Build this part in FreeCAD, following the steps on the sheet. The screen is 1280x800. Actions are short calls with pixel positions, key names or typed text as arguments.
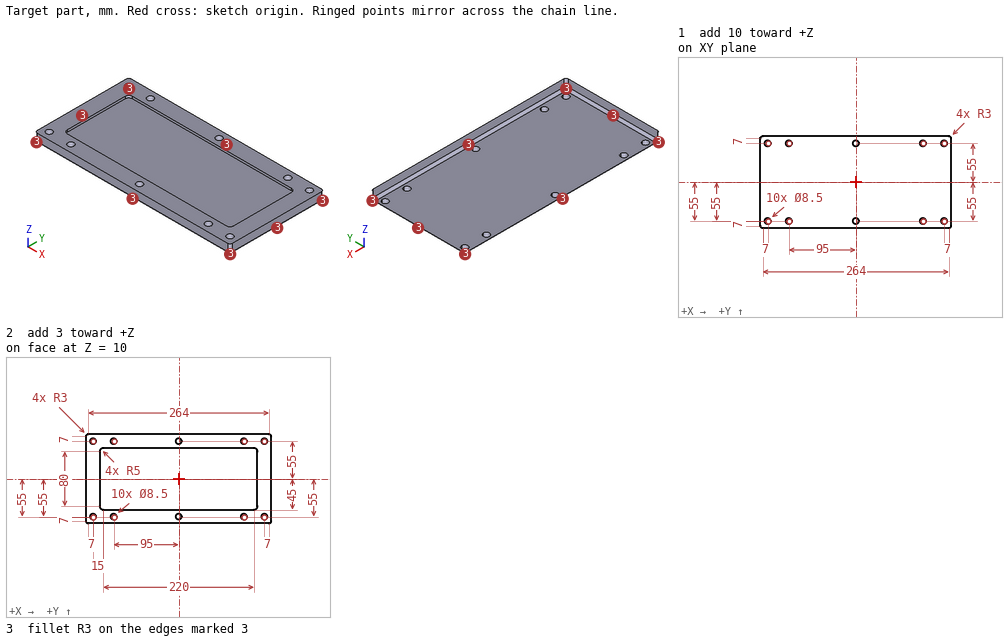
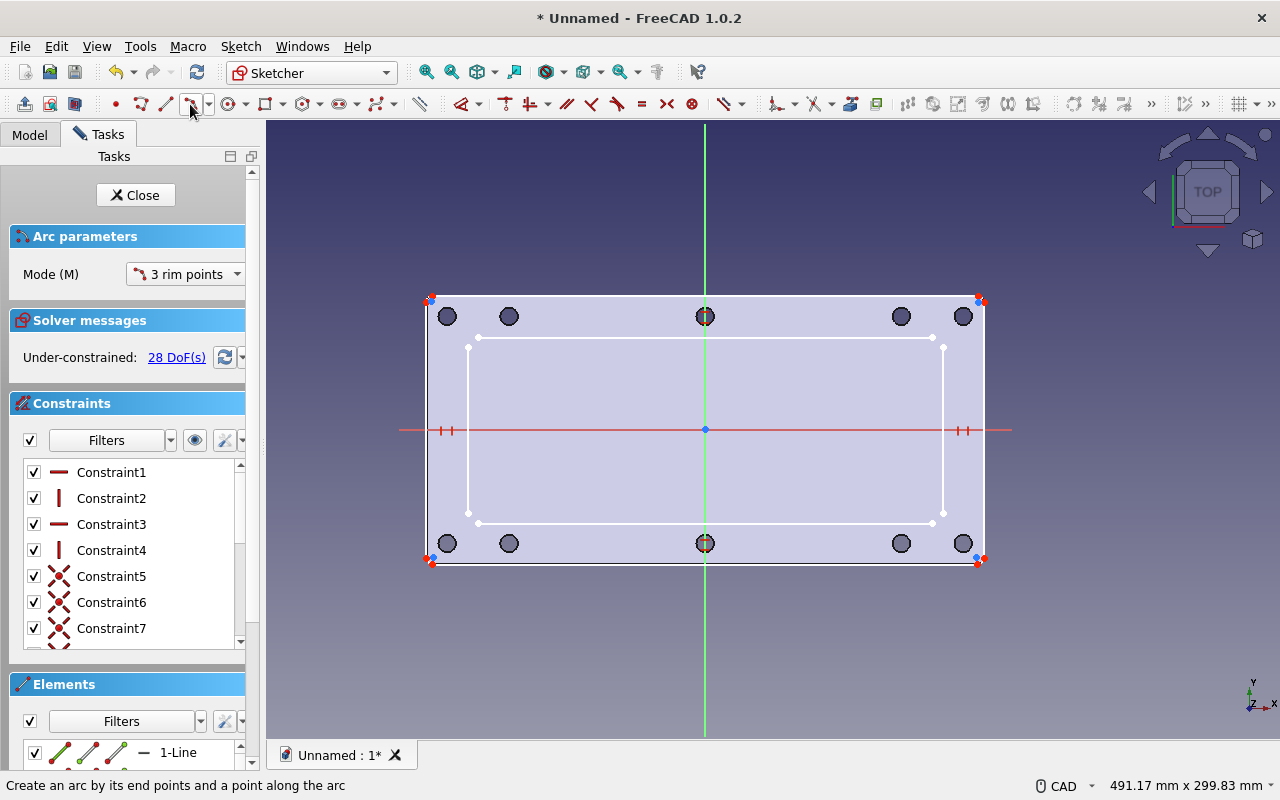
click(478, 524)
click(468, 514)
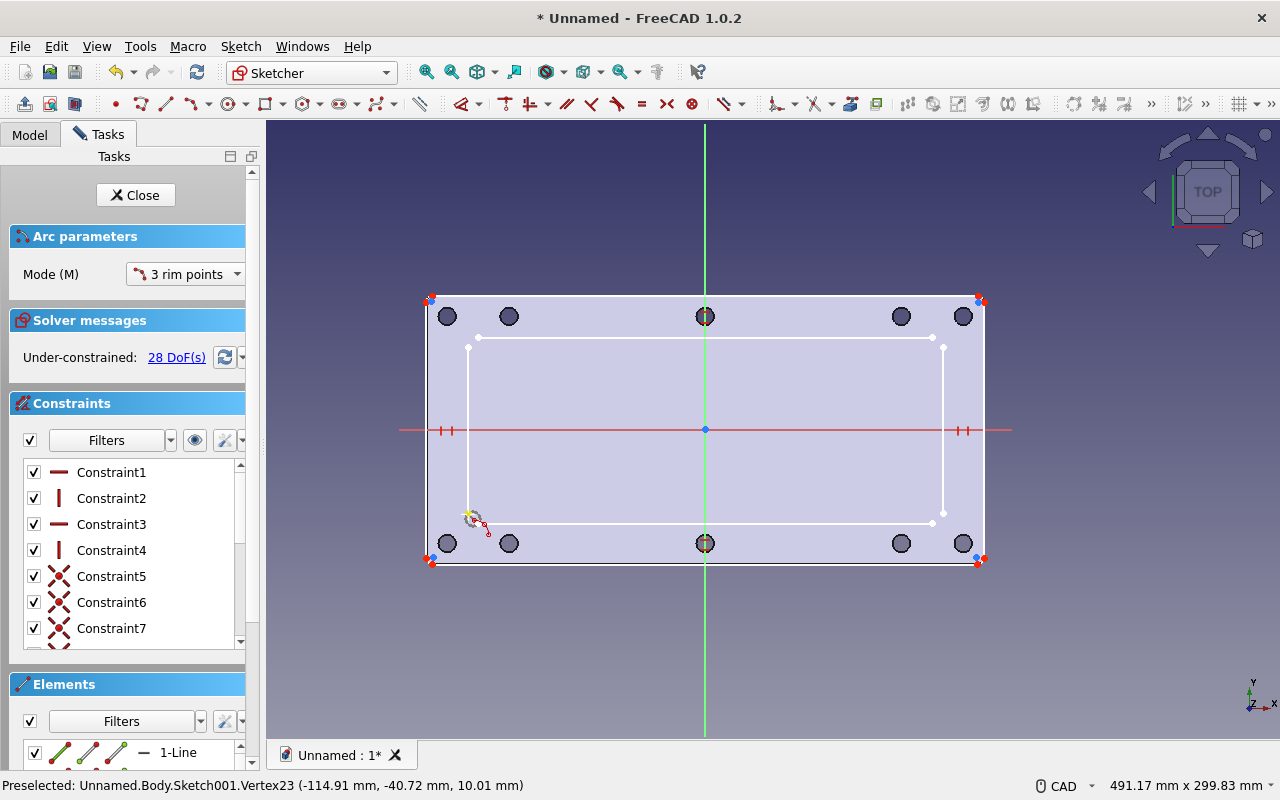
scroll(471, 520, up, 9)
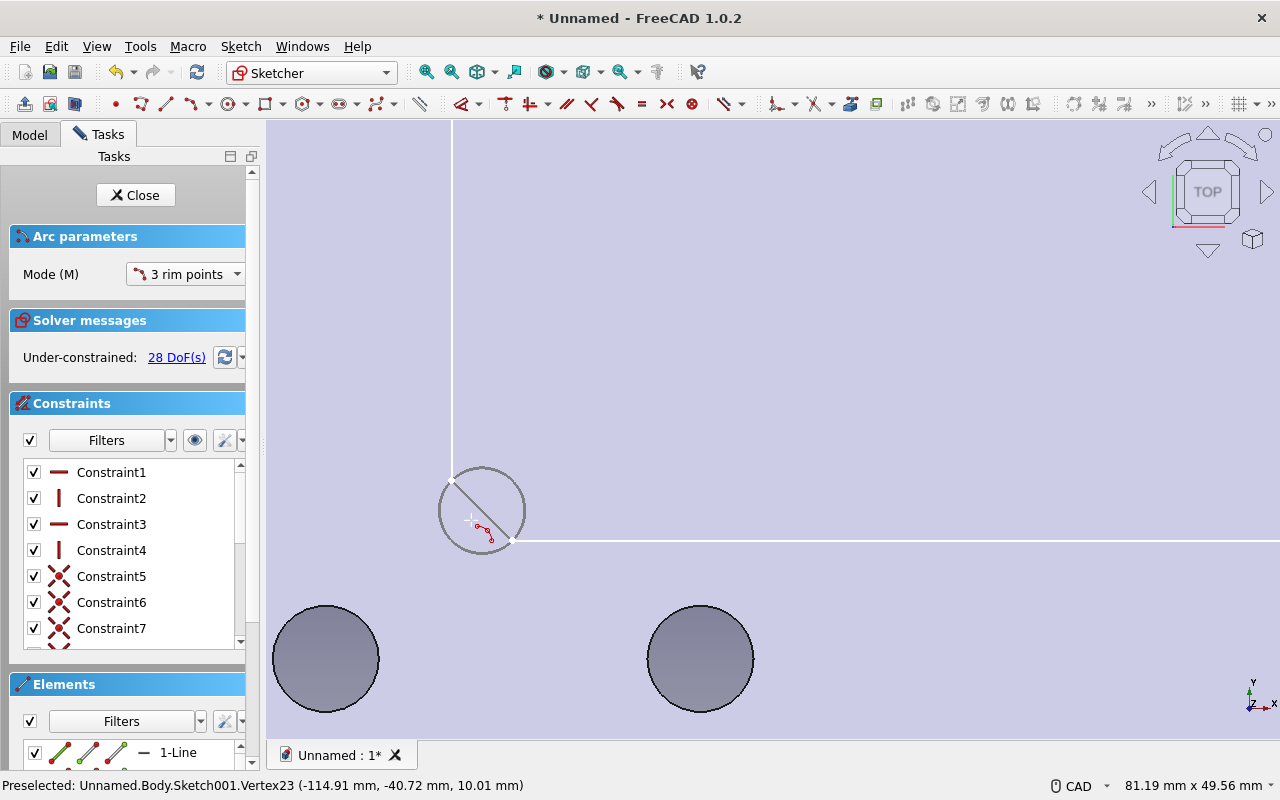
click(469, 516)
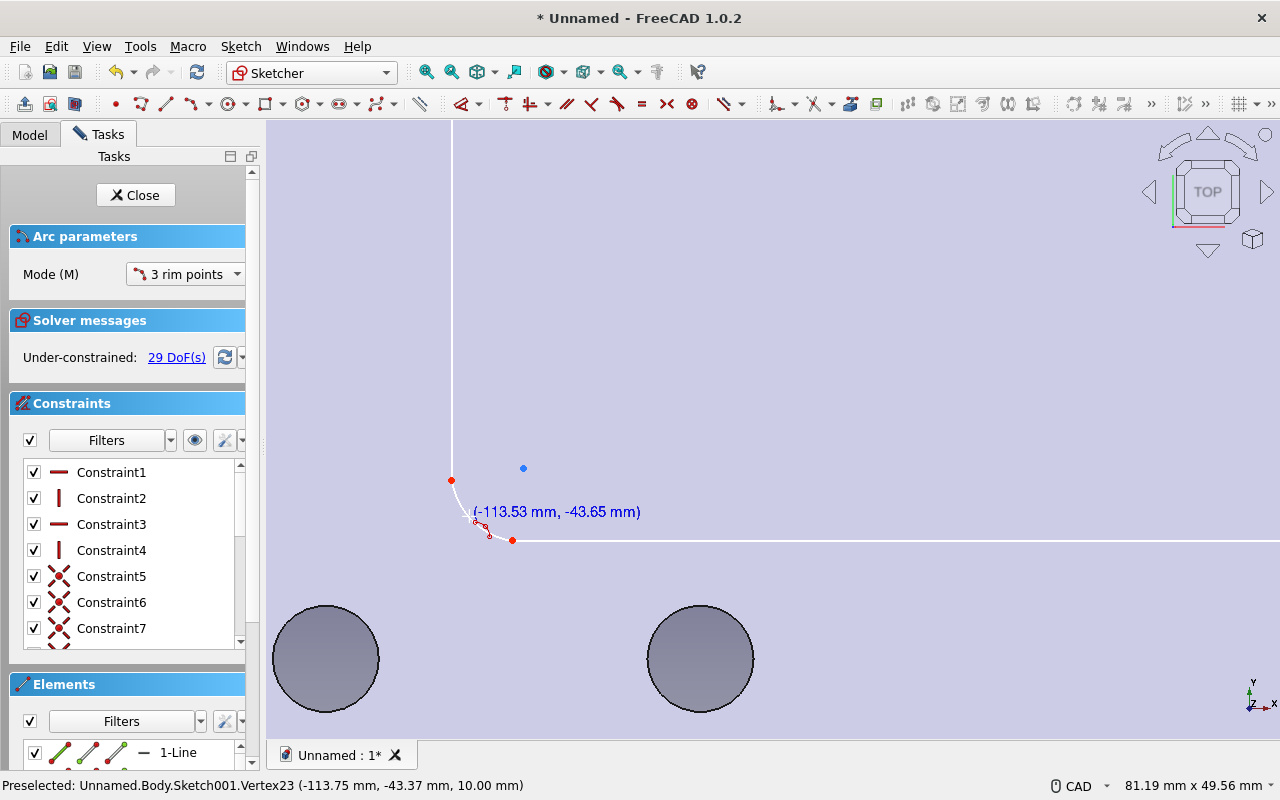
scroll(470, 520, down, 9)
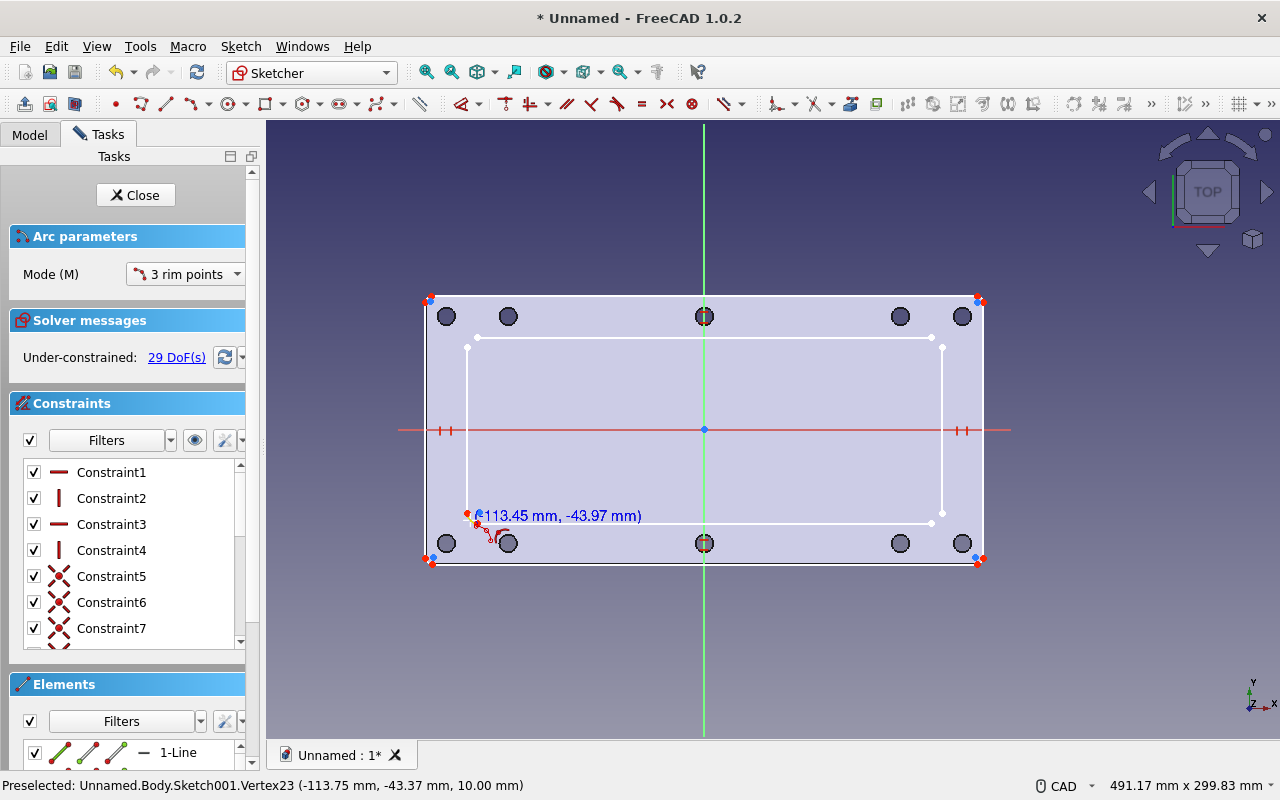
click(467, 348)
click(477, 338)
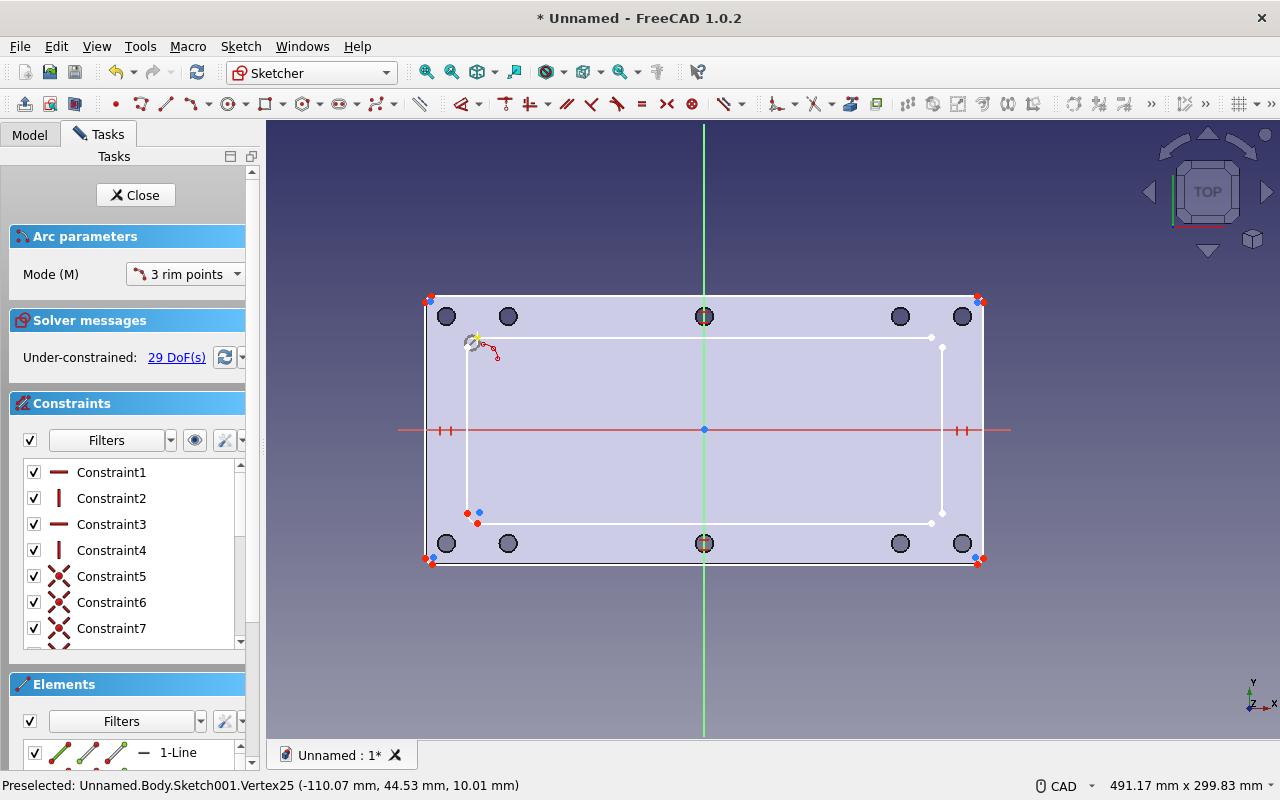
scroll(470, 340, up, 9)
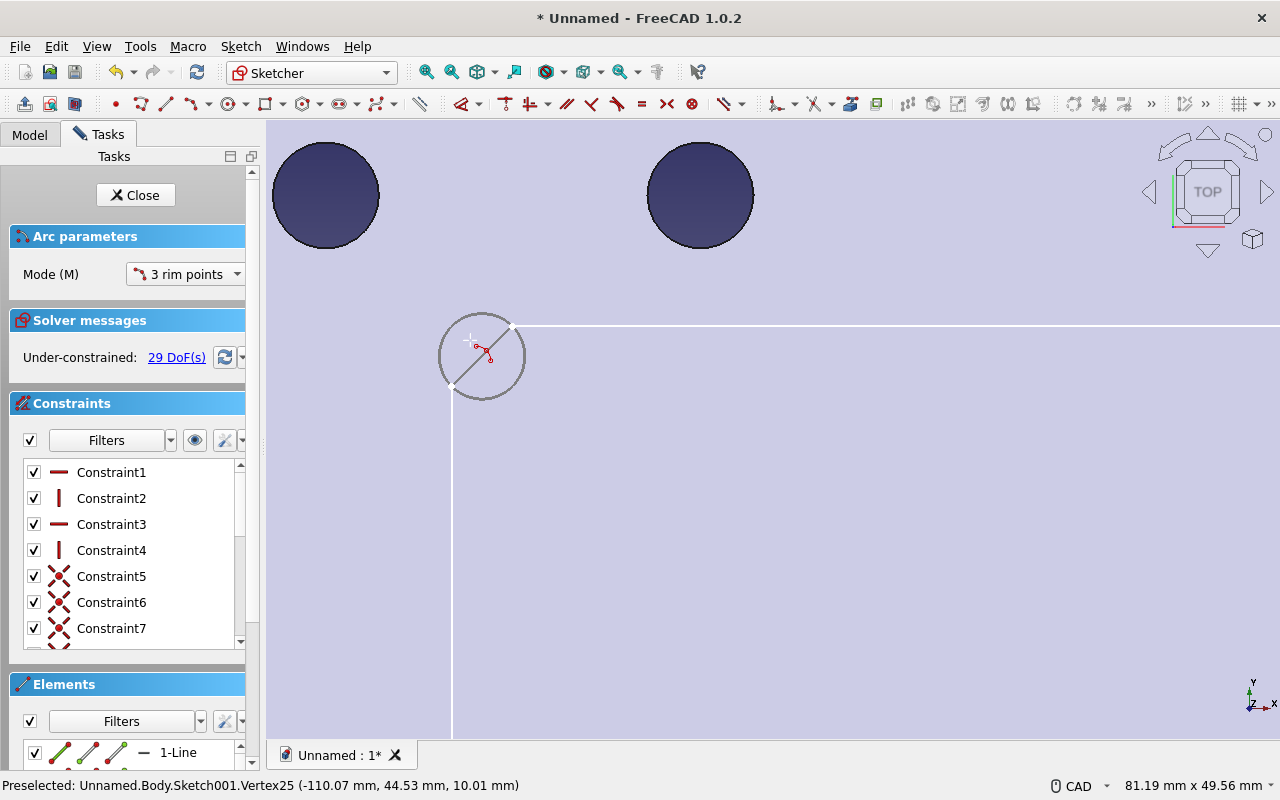
click(469, 339)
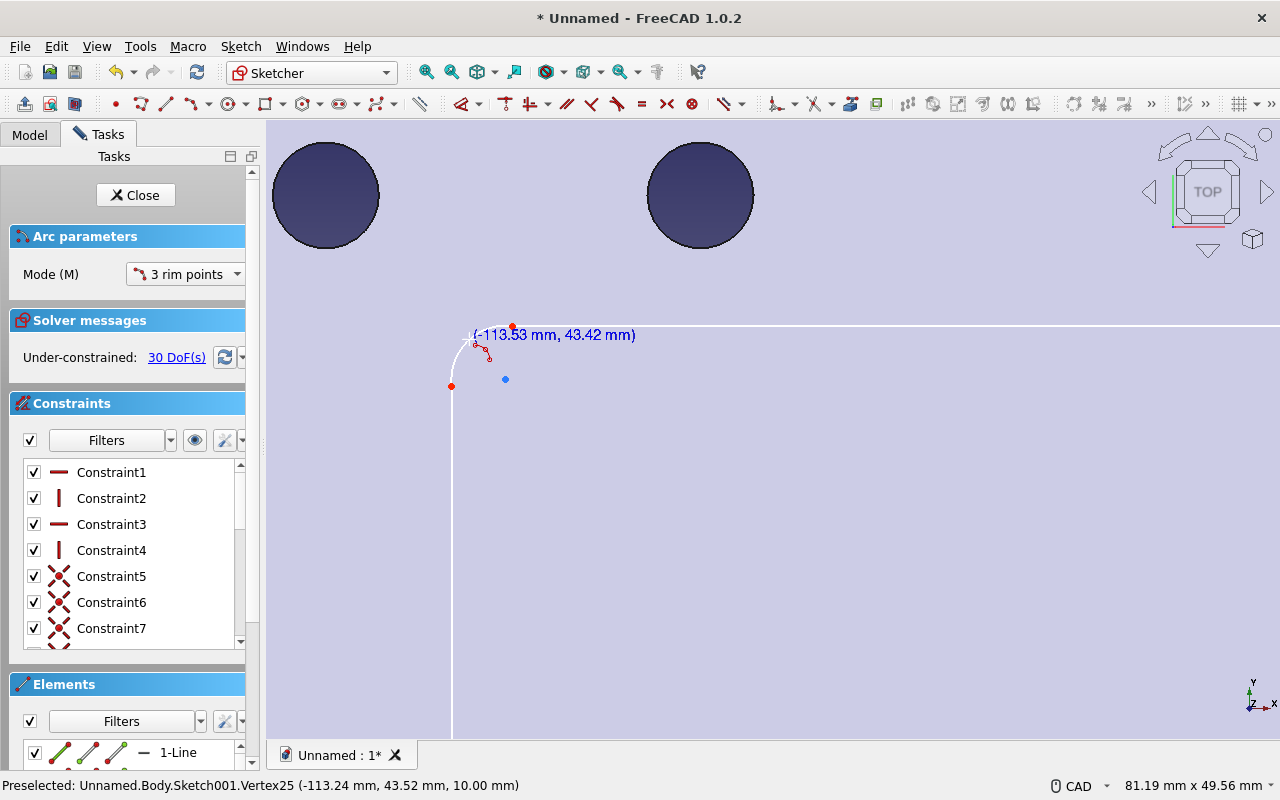
scroll(470, 340, down, 9)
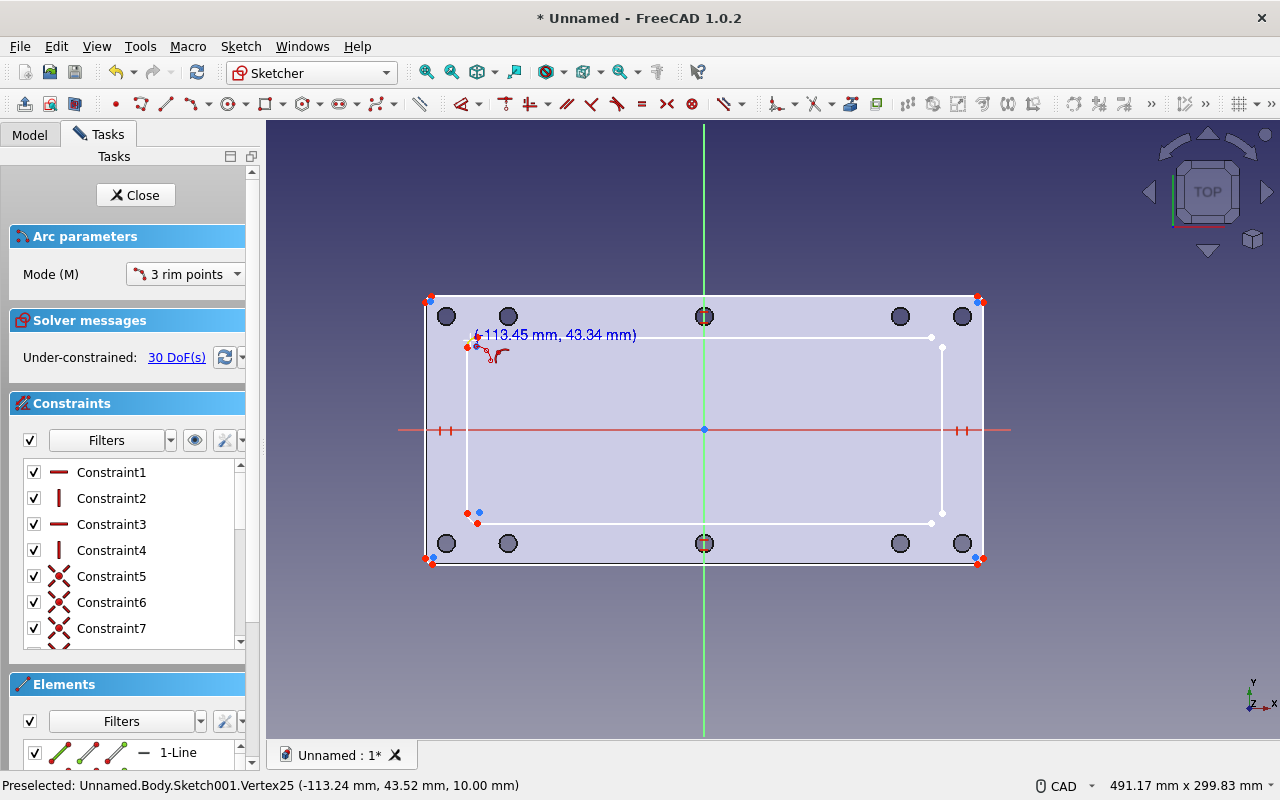
click(931, 338)
click(942, 348)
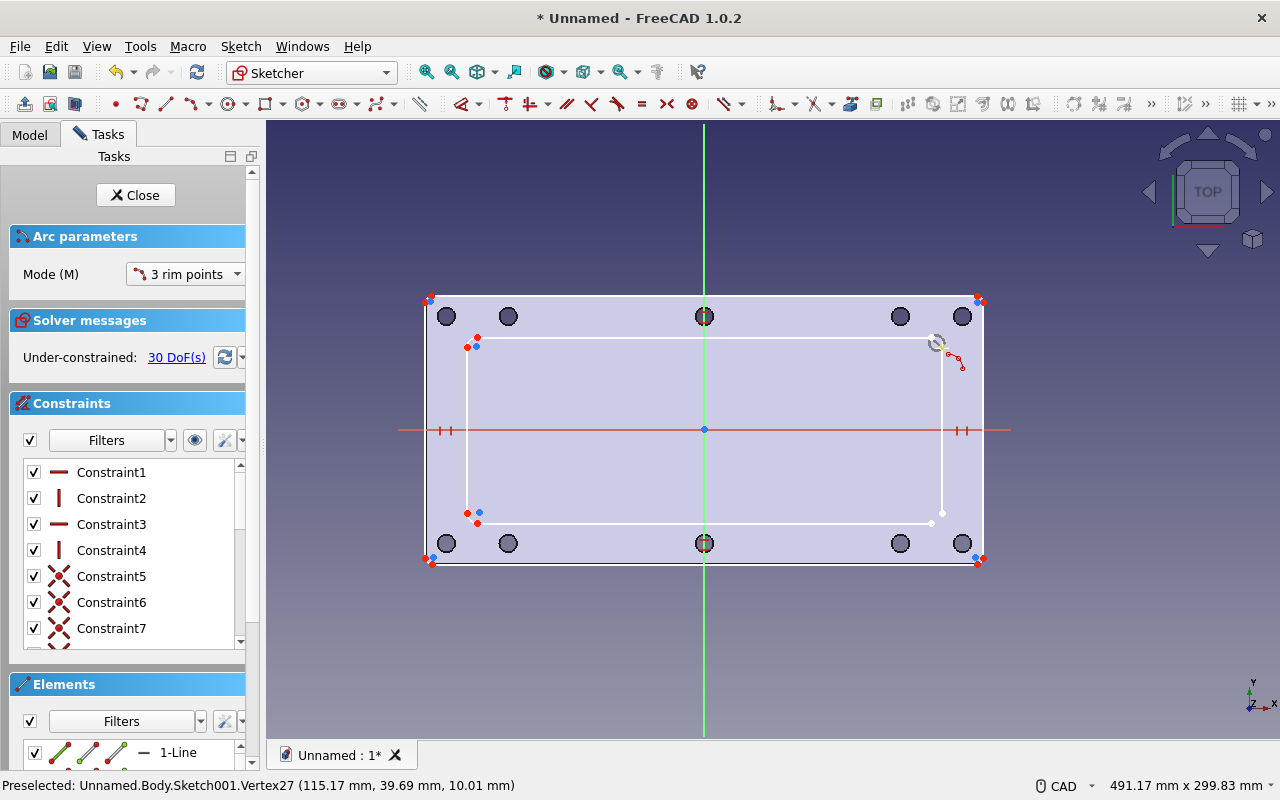
scroll(939, 340, up, 9)